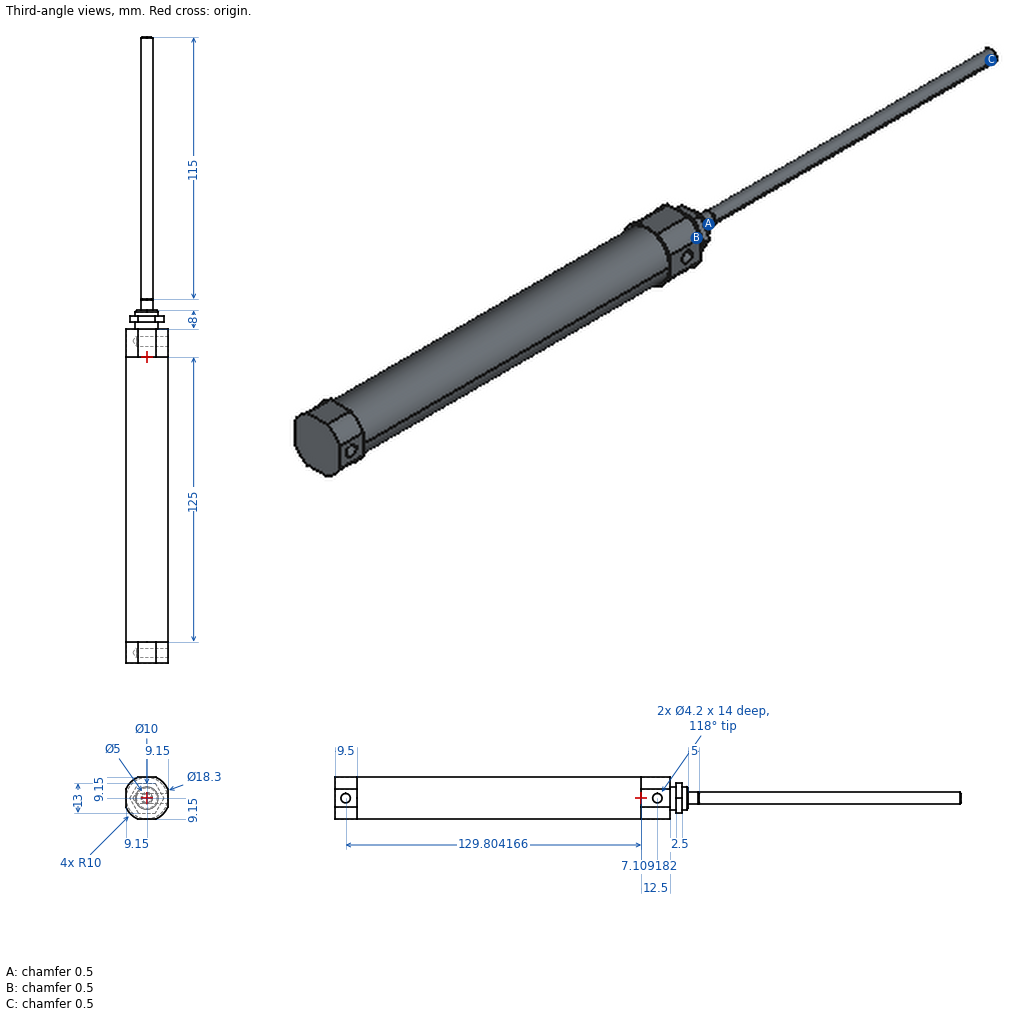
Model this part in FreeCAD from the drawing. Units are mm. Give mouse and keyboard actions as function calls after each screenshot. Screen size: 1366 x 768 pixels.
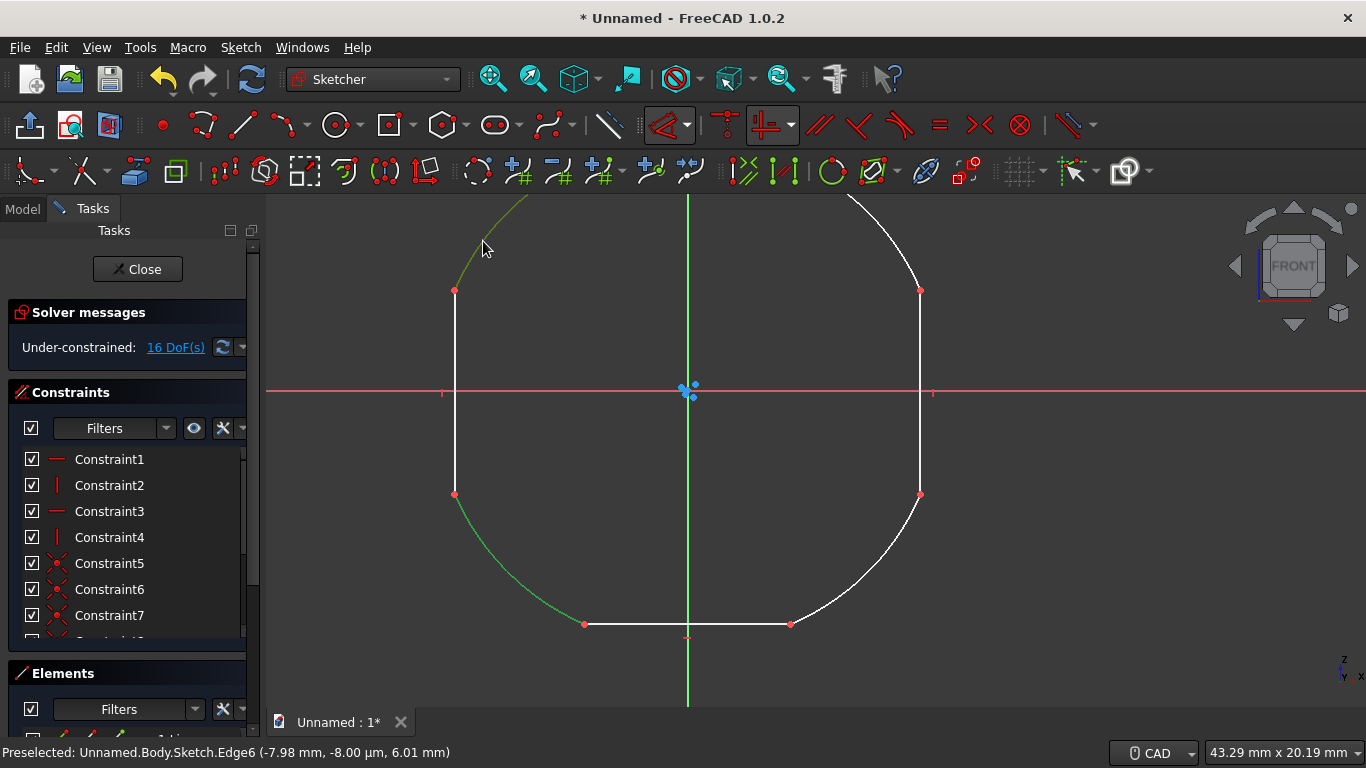
key(c)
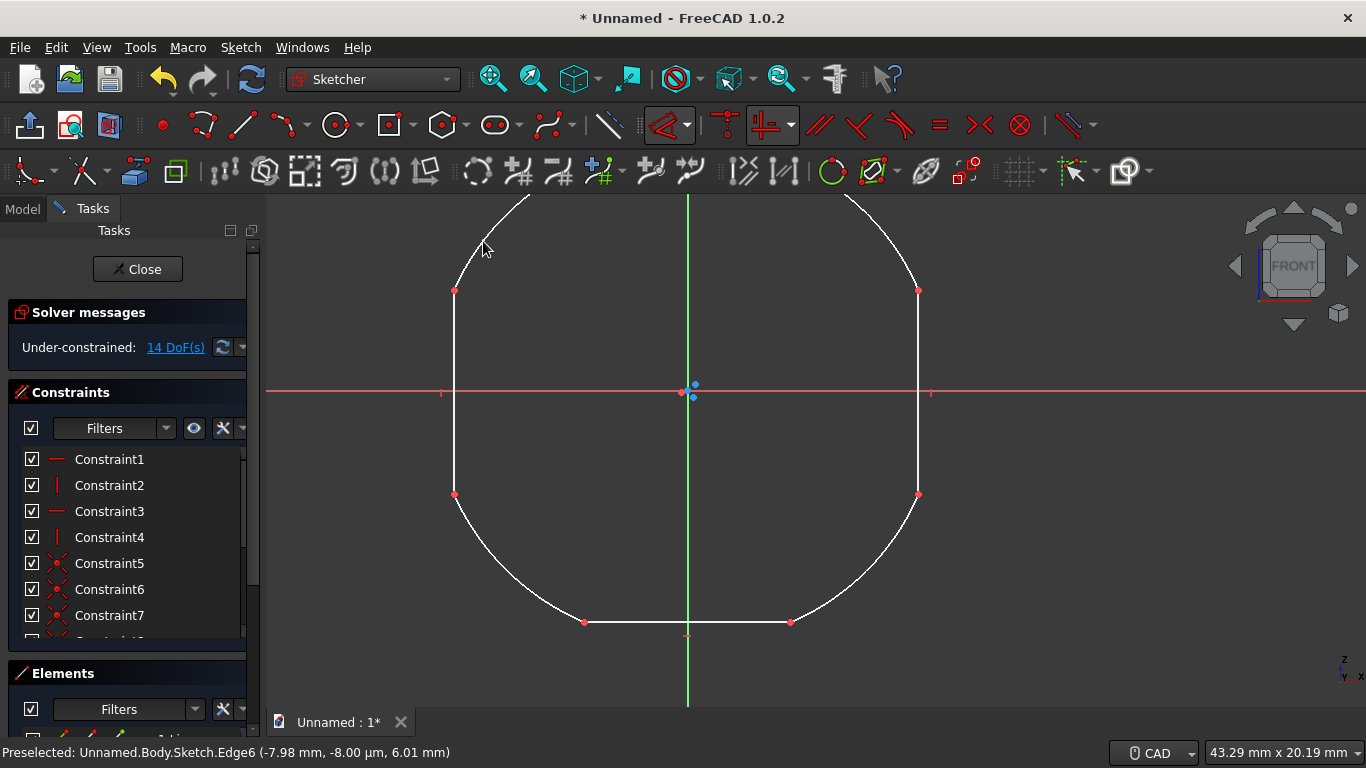
click(483, 543)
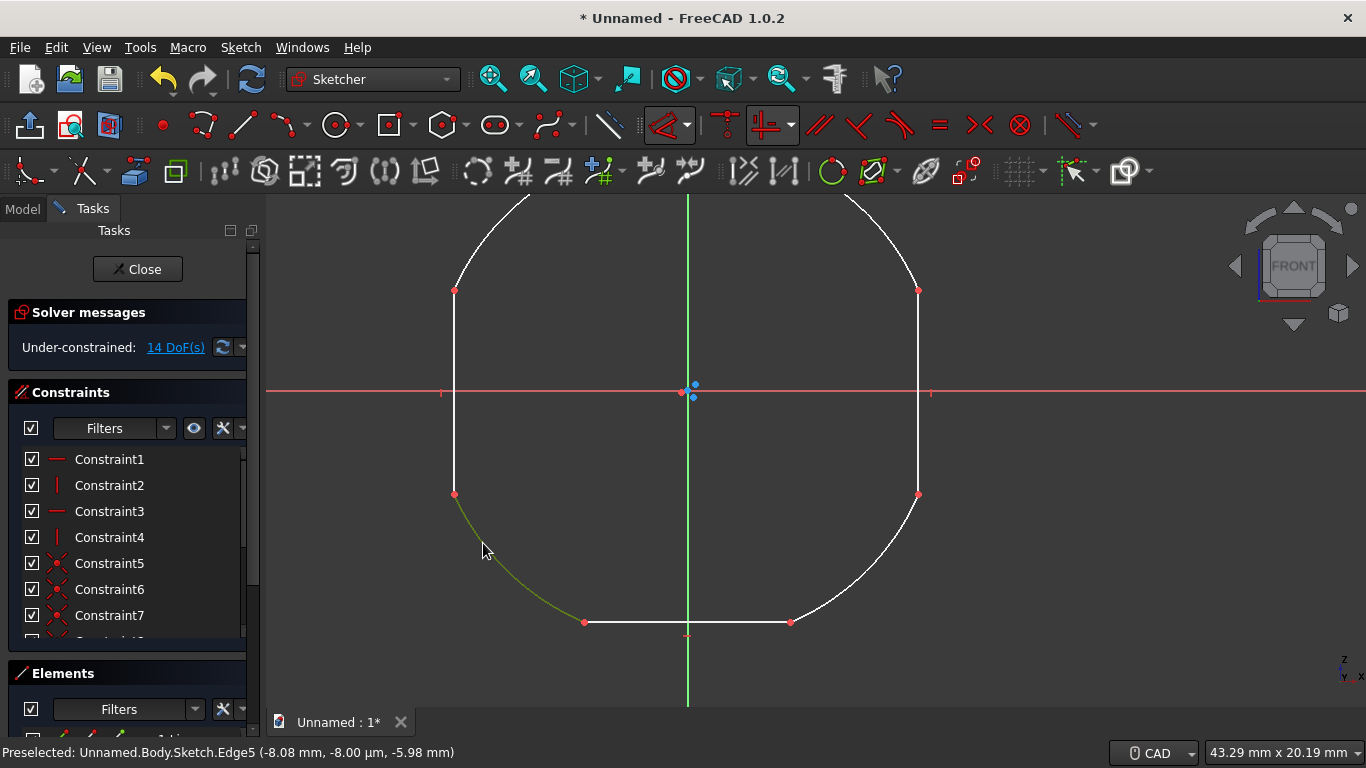
click(891, 242)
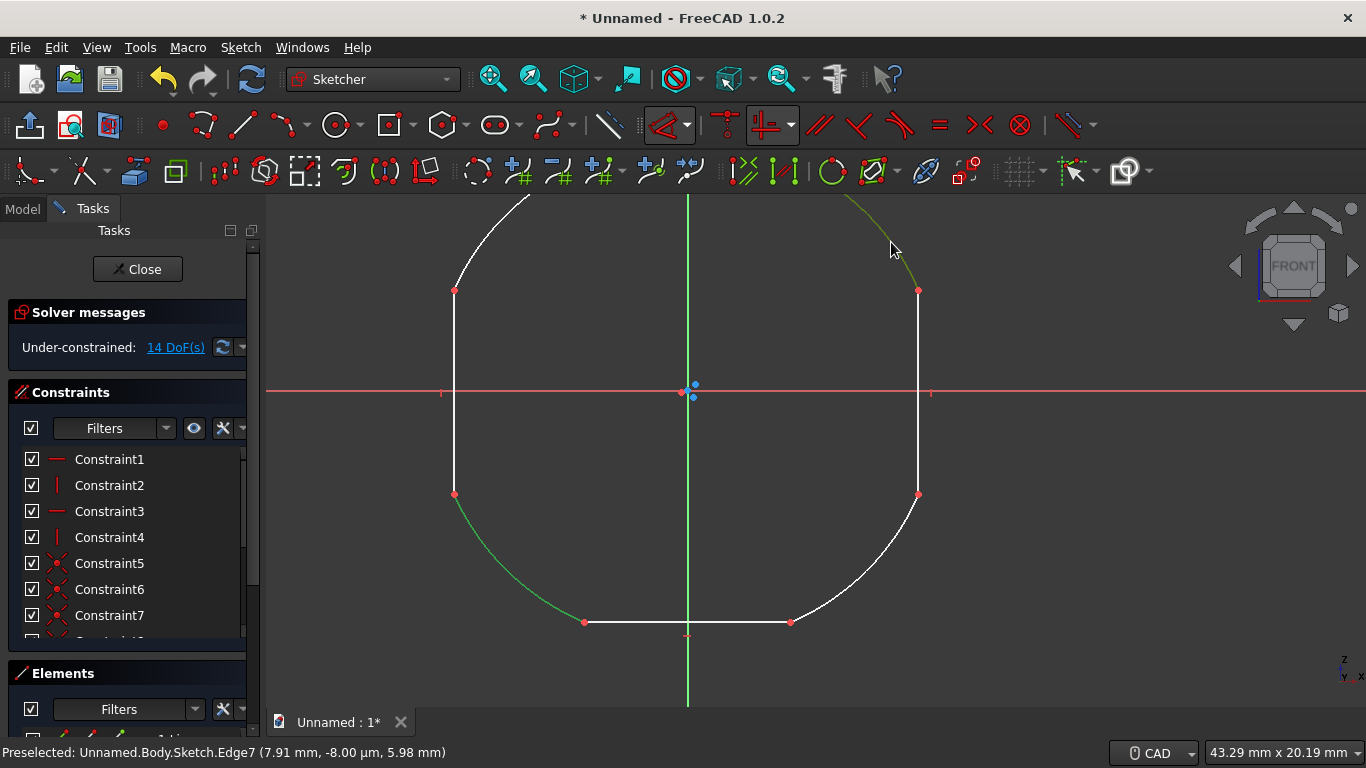
key(c)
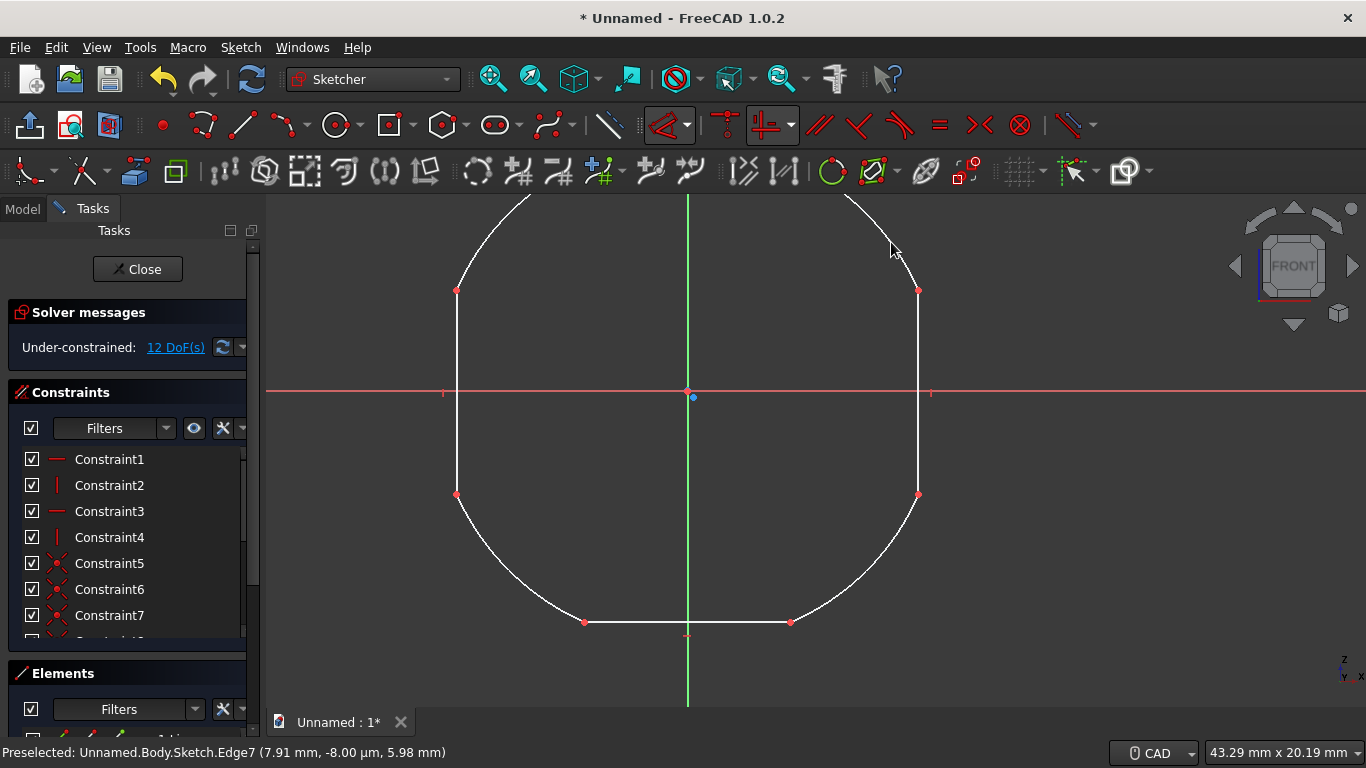
click(485, 542)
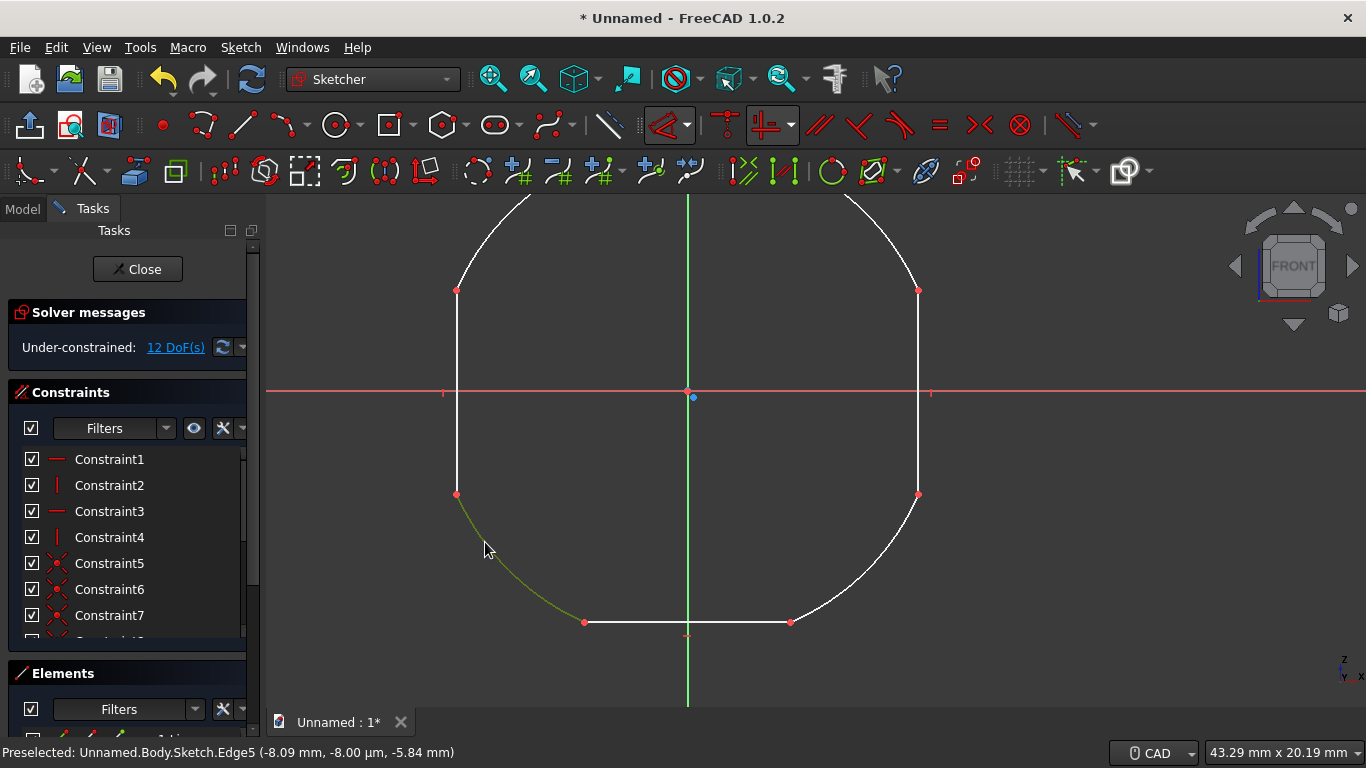
click(839, 595)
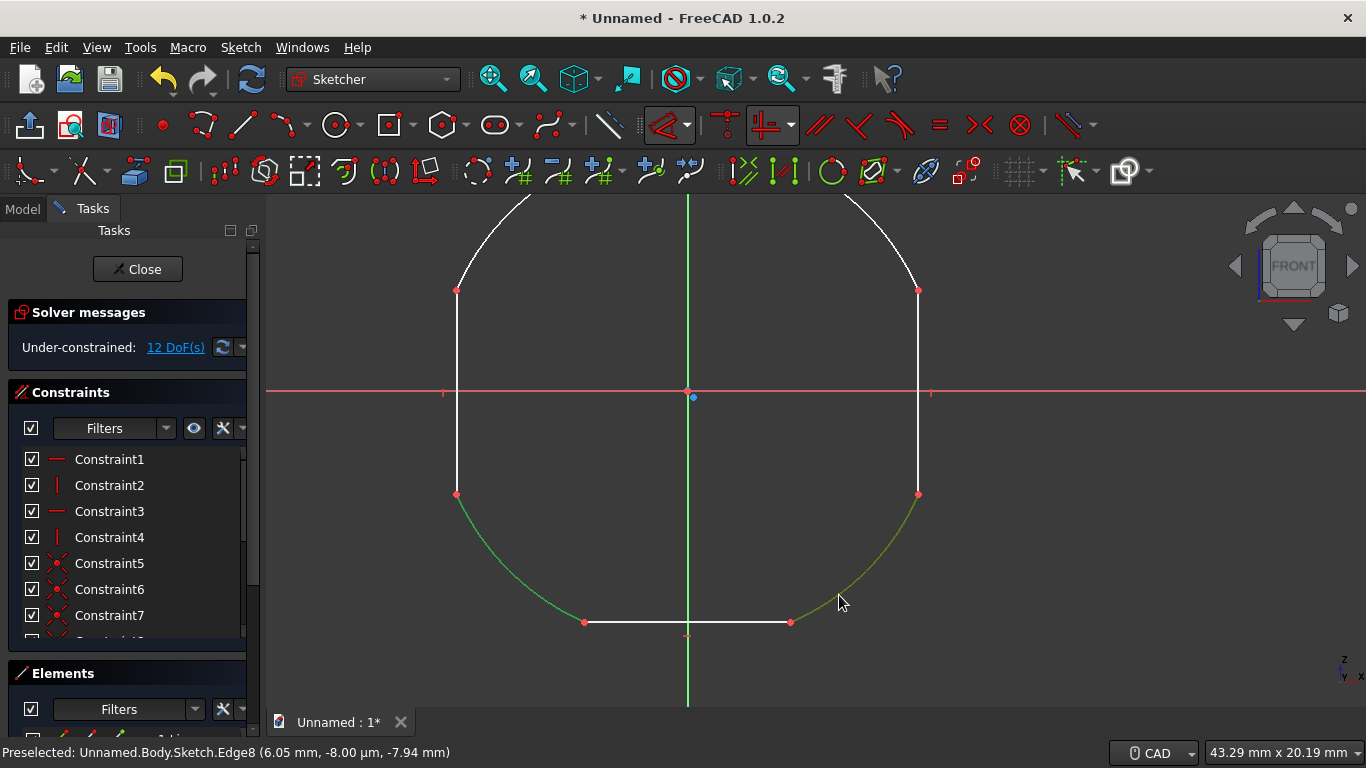
key(c)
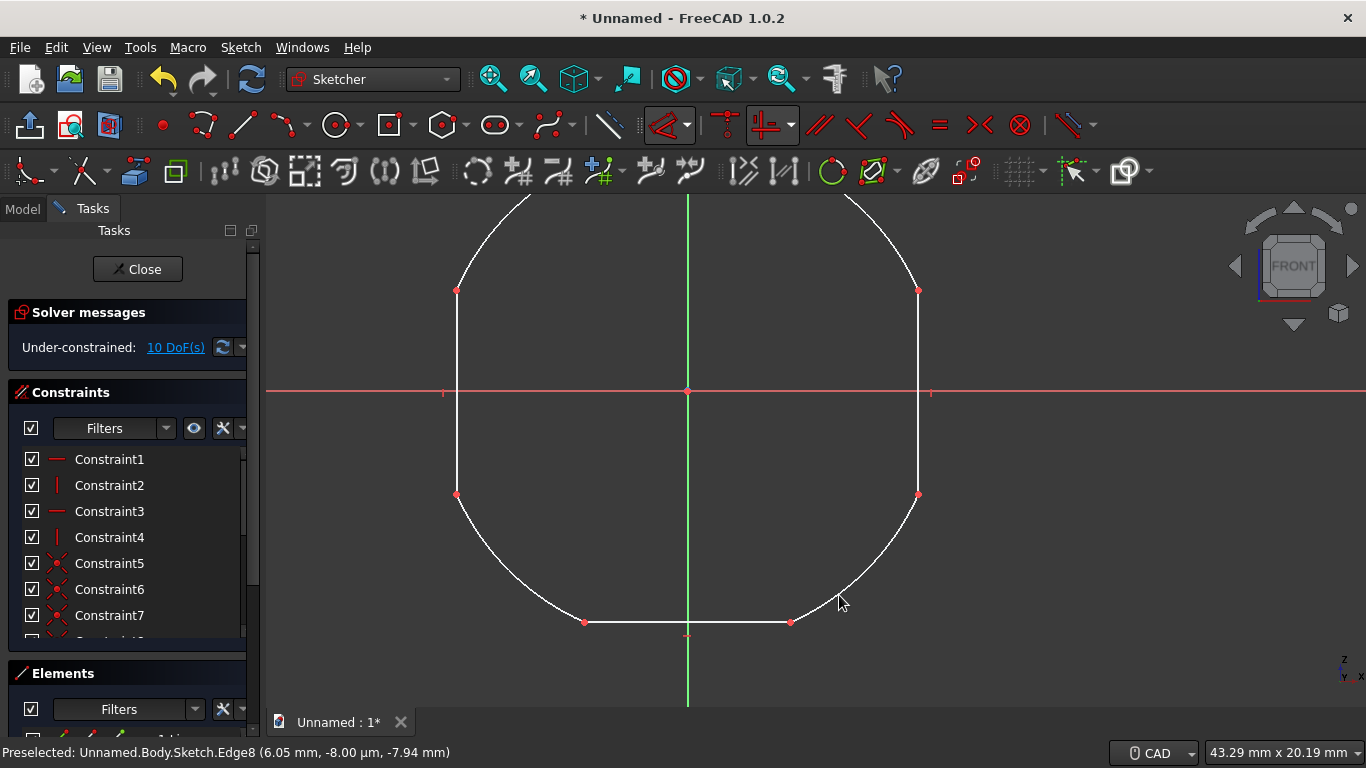
drag(677, 381, 698, 402)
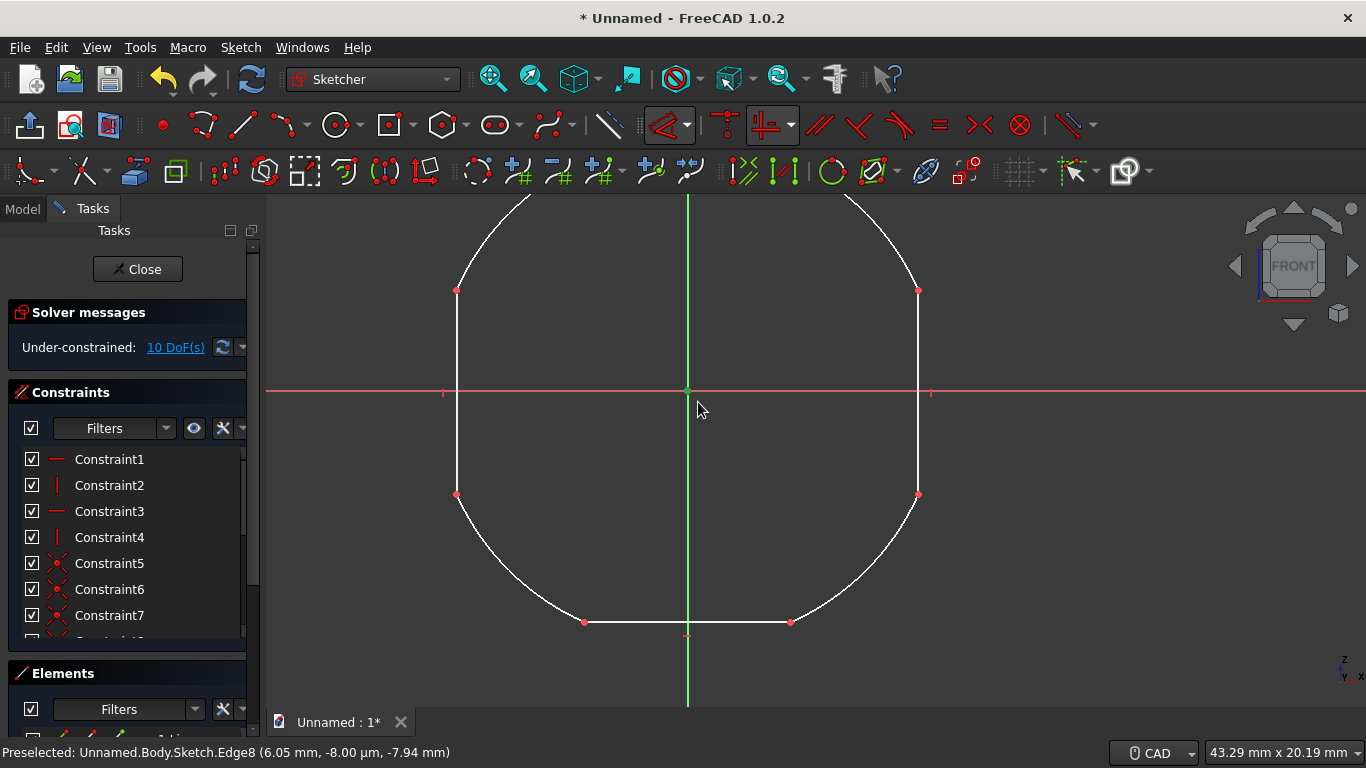
key(c)